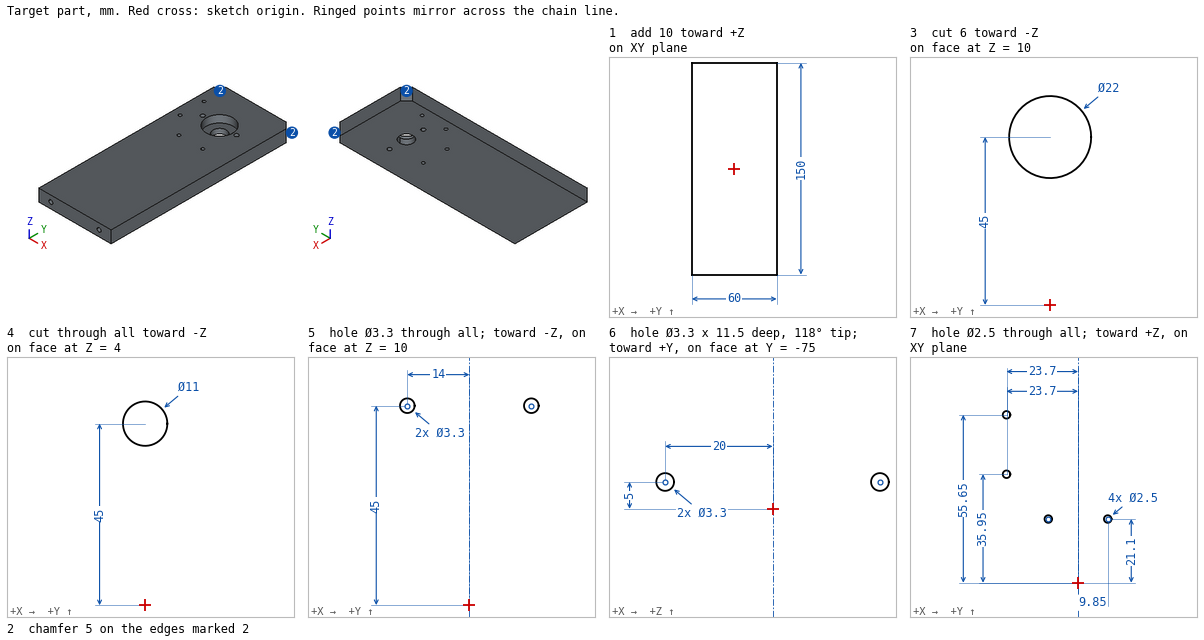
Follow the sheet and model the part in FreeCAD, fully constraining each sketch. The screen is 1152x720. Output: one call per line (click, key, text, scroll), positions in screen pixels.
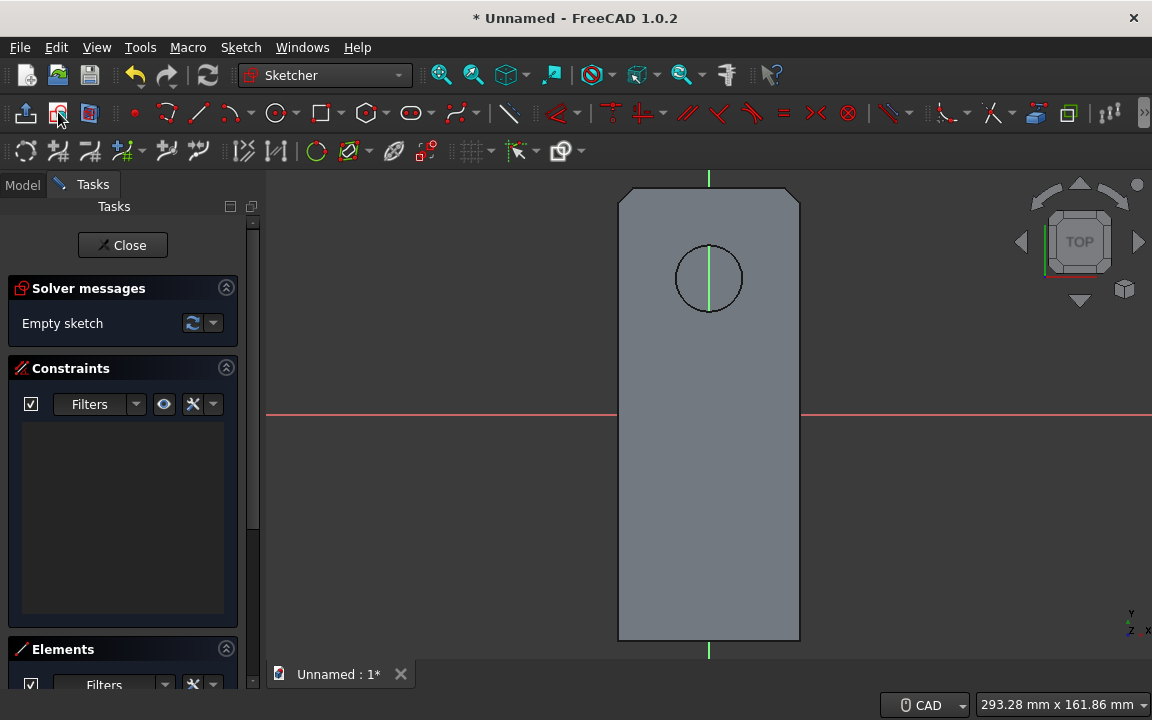
click(90, 114)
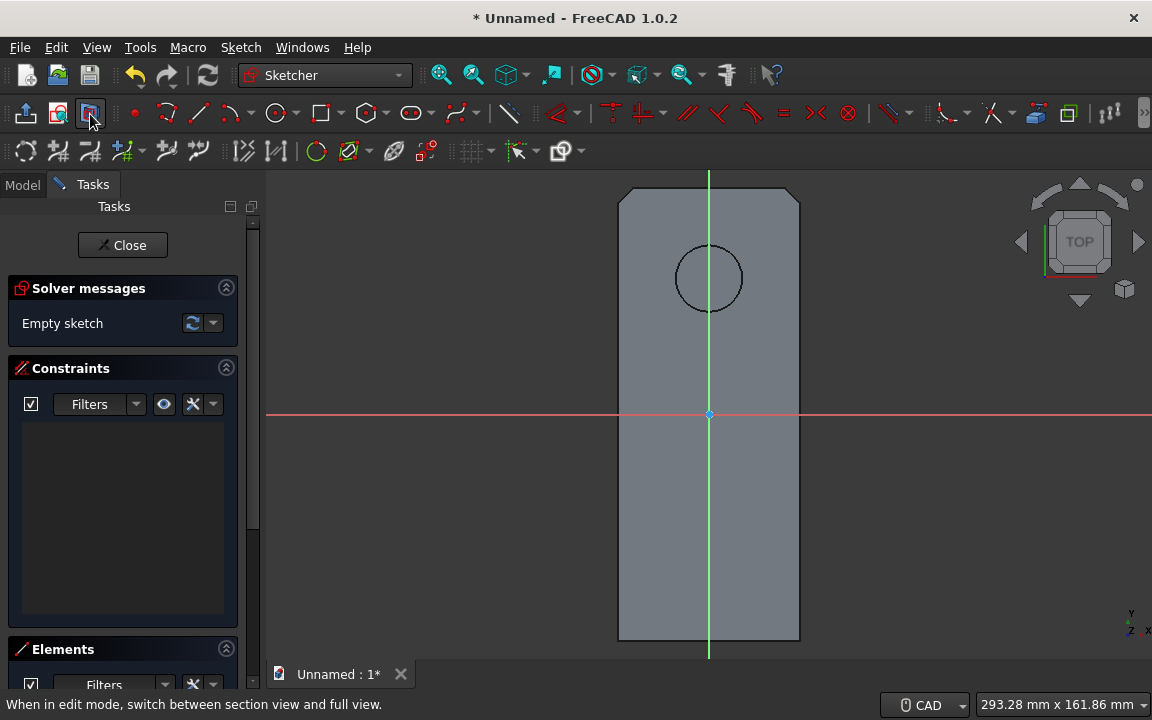
scroll(718, 262, up, 11)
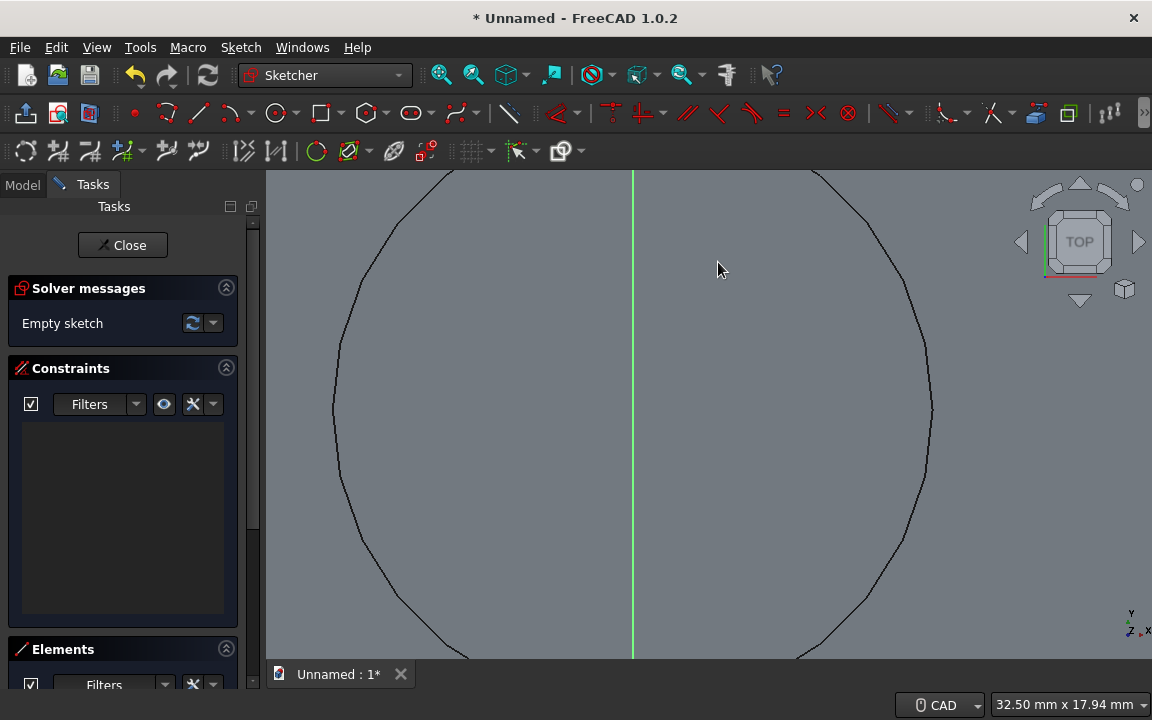
click(276, 114)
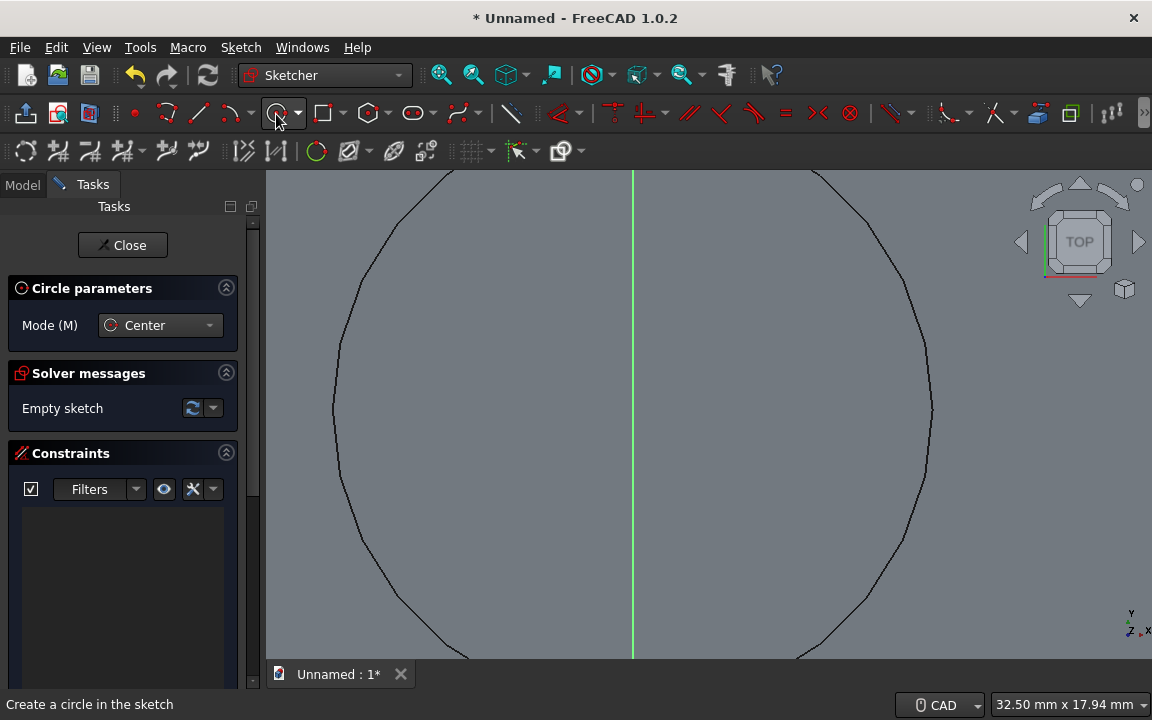
click(633, 410)
click(739, 304)
key(Escape)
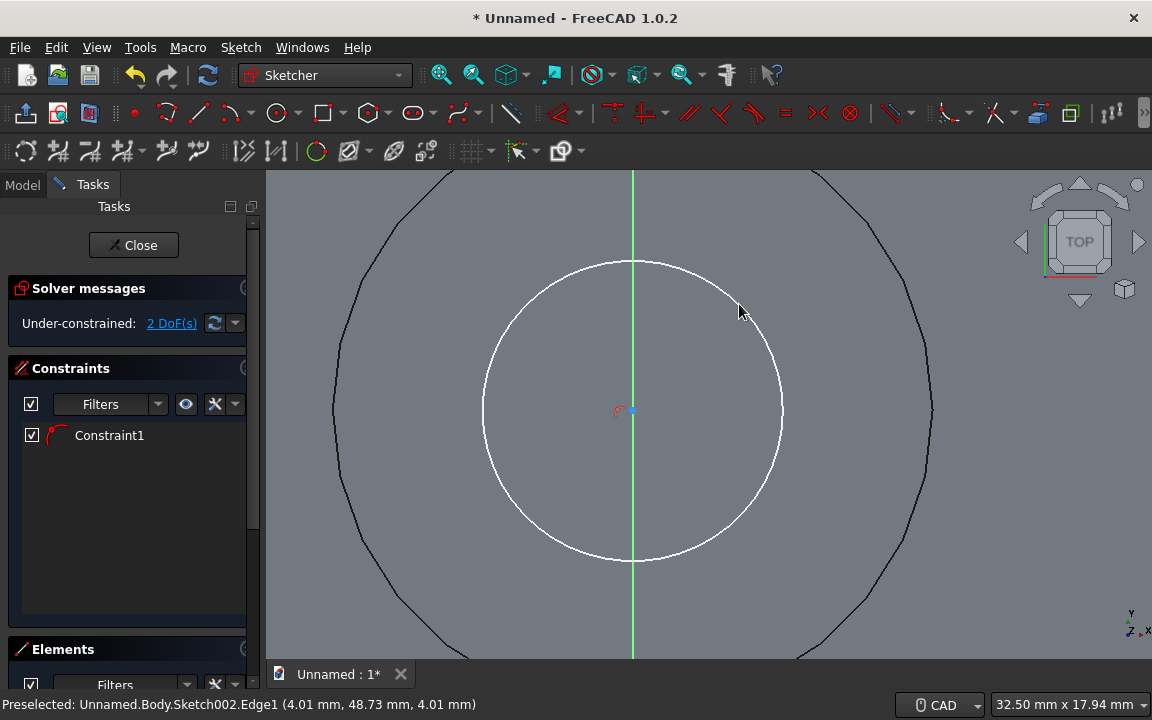
click(558, 114)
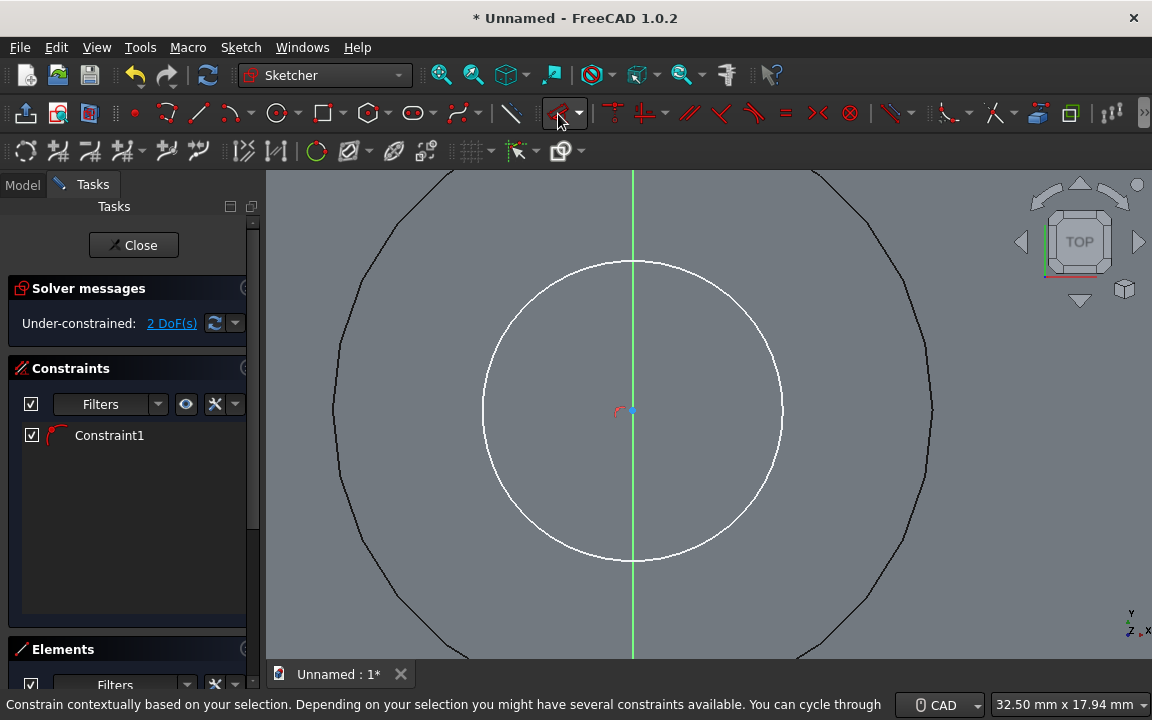
click(739, 305)
click(762, 282)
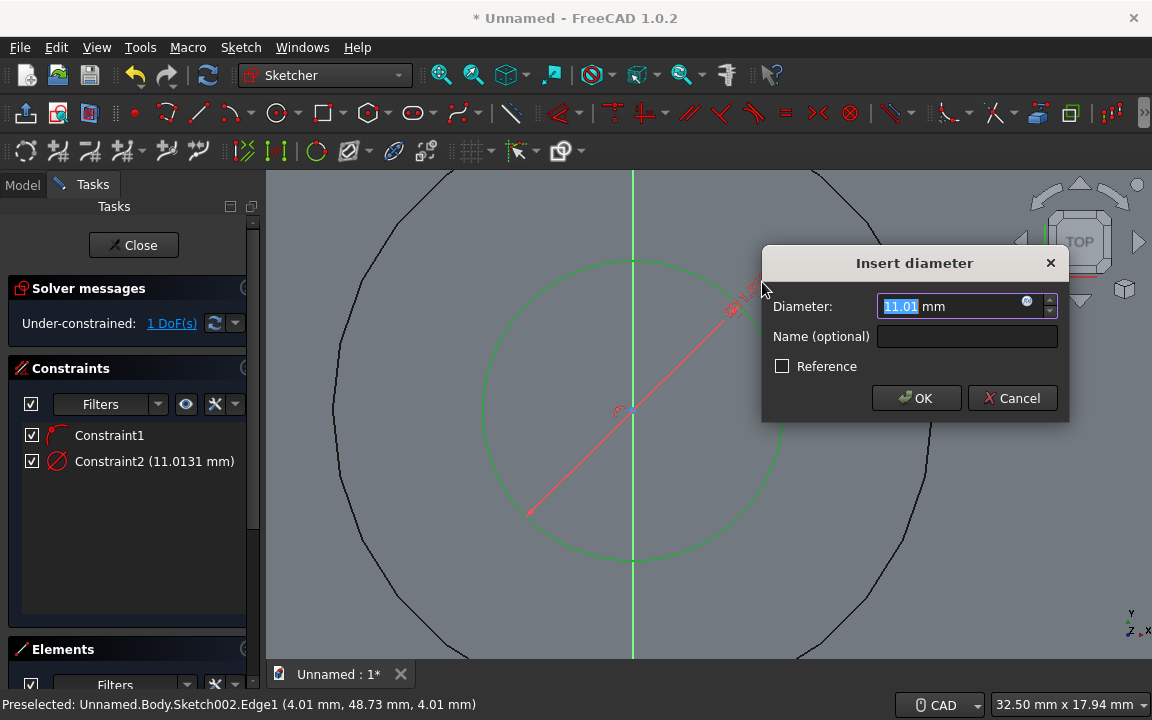
text(11)
key(Return)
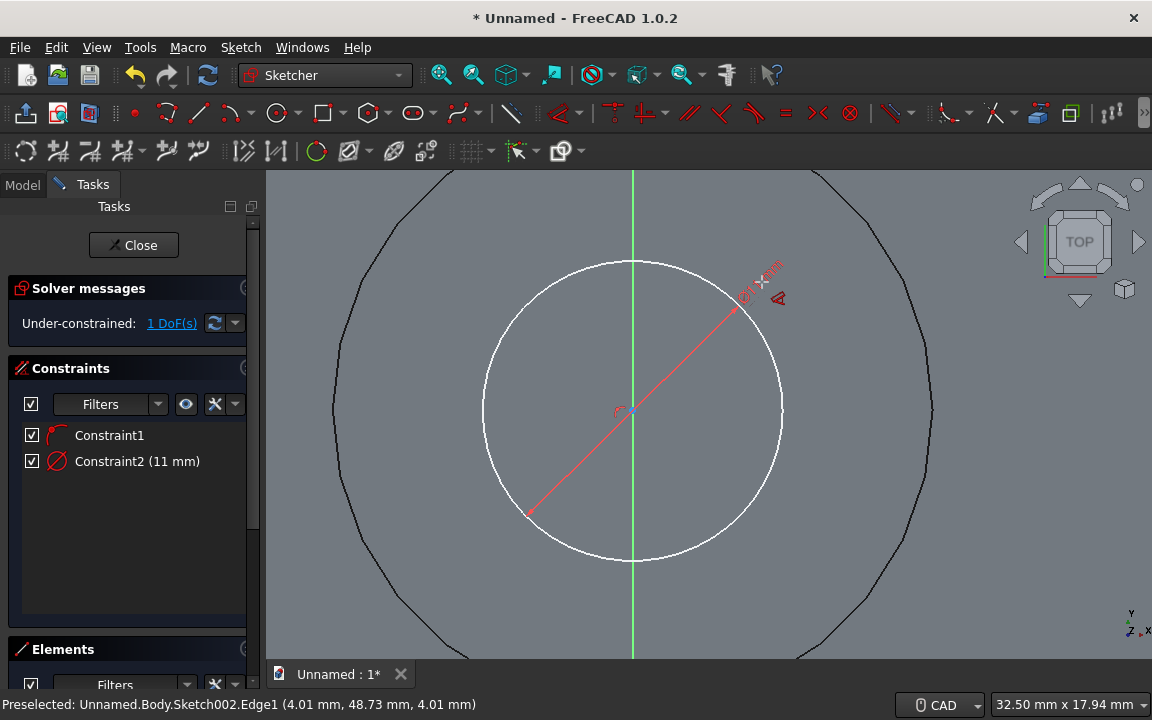
click(633, 411)
click(667, 521)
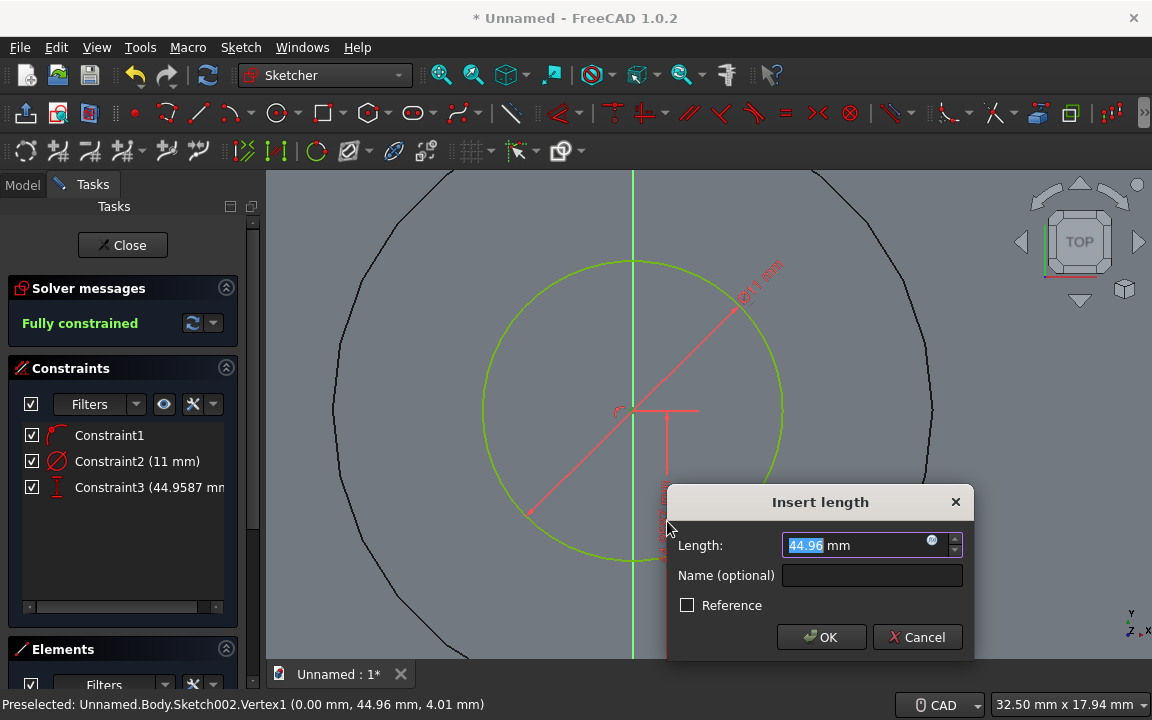
text(45)
key(Return)
key(Escape)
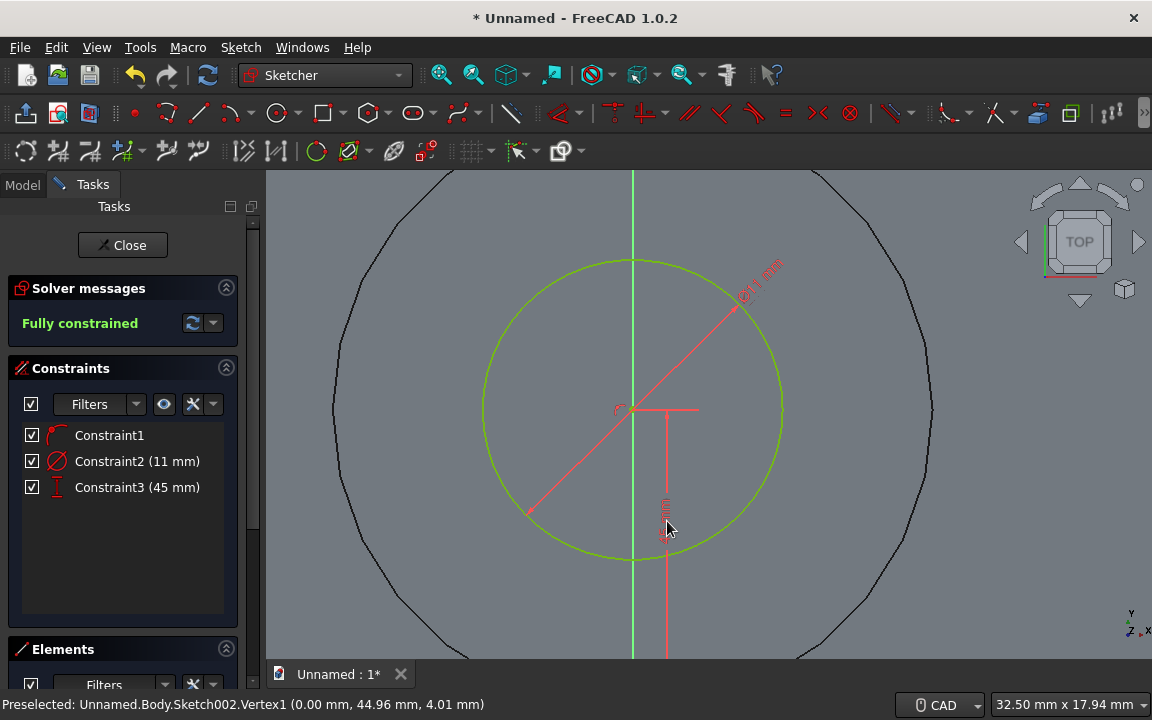
click(123, 245)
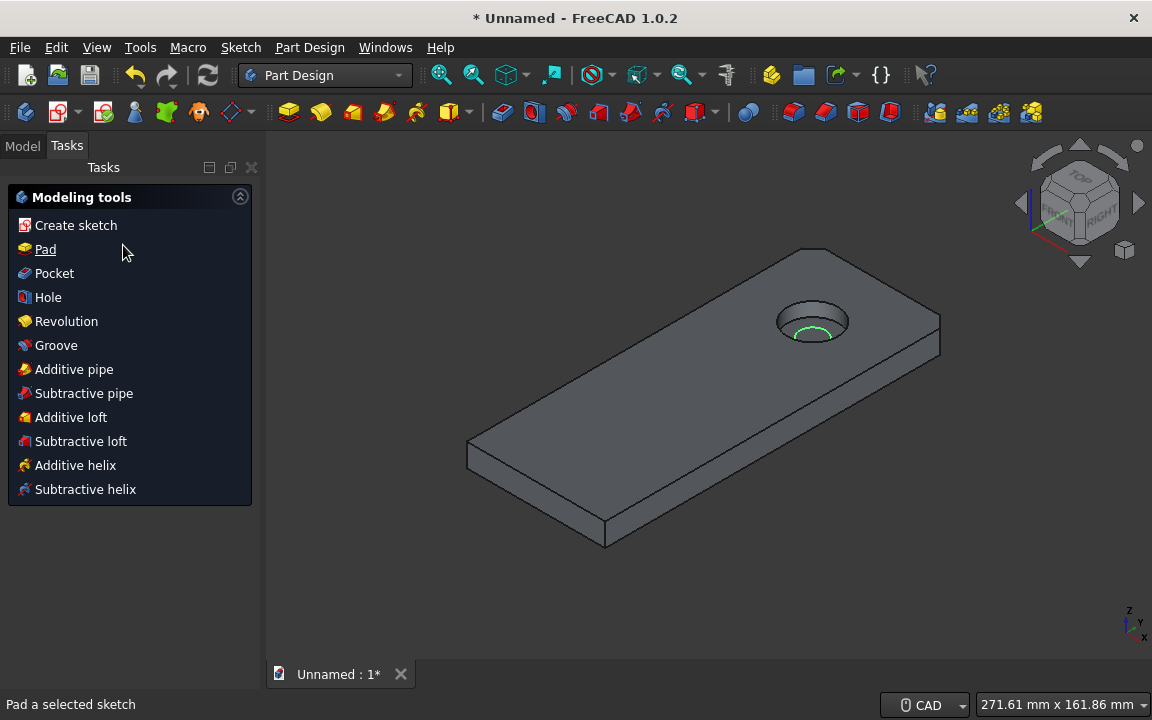
click(504, 112)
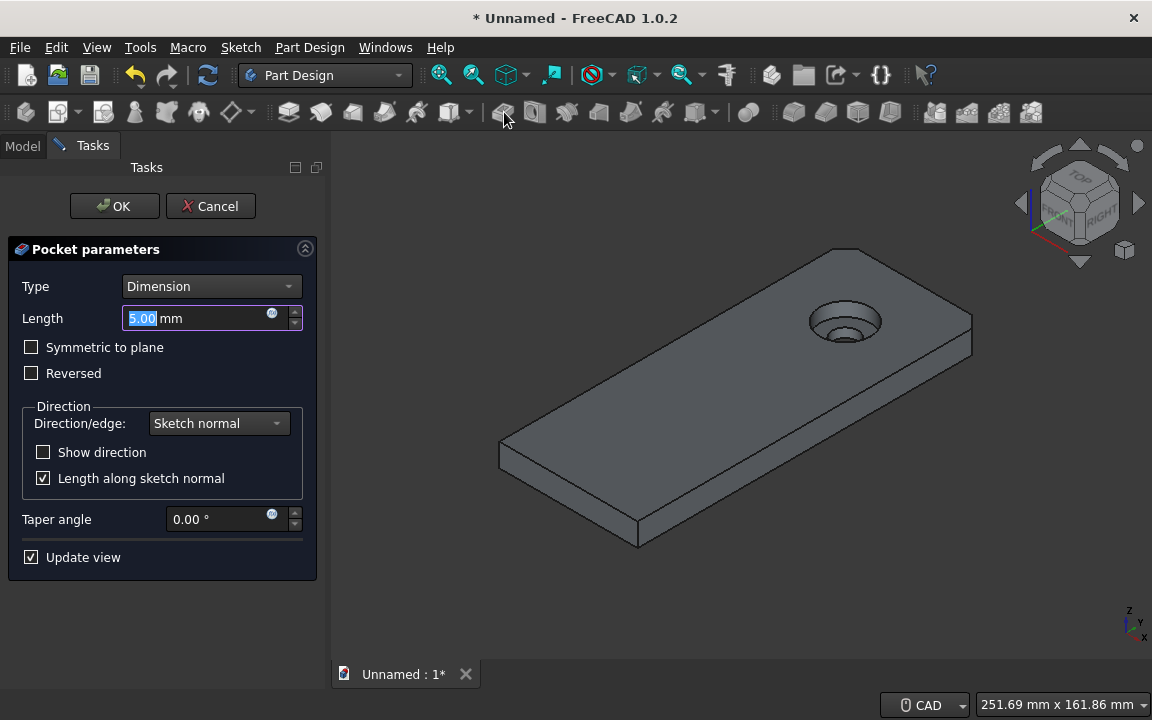
click(212, 286)